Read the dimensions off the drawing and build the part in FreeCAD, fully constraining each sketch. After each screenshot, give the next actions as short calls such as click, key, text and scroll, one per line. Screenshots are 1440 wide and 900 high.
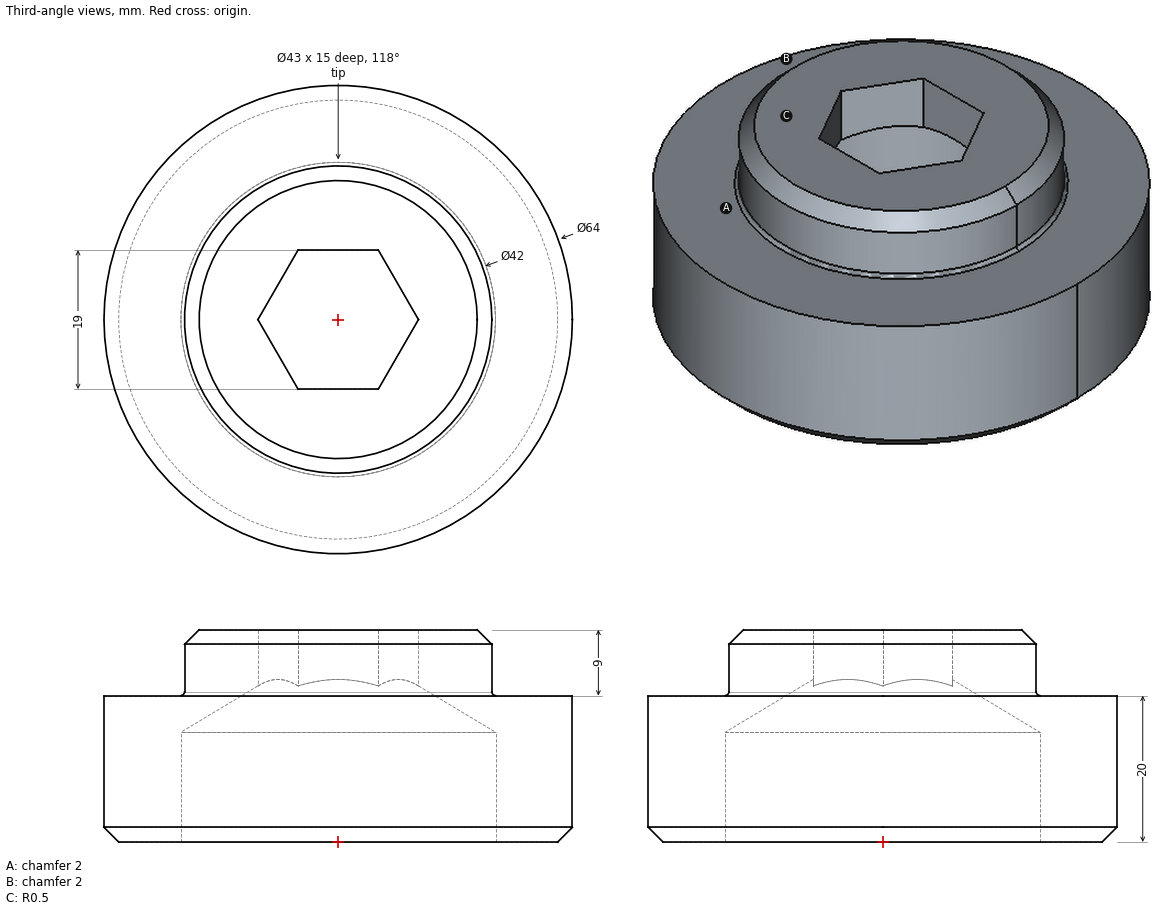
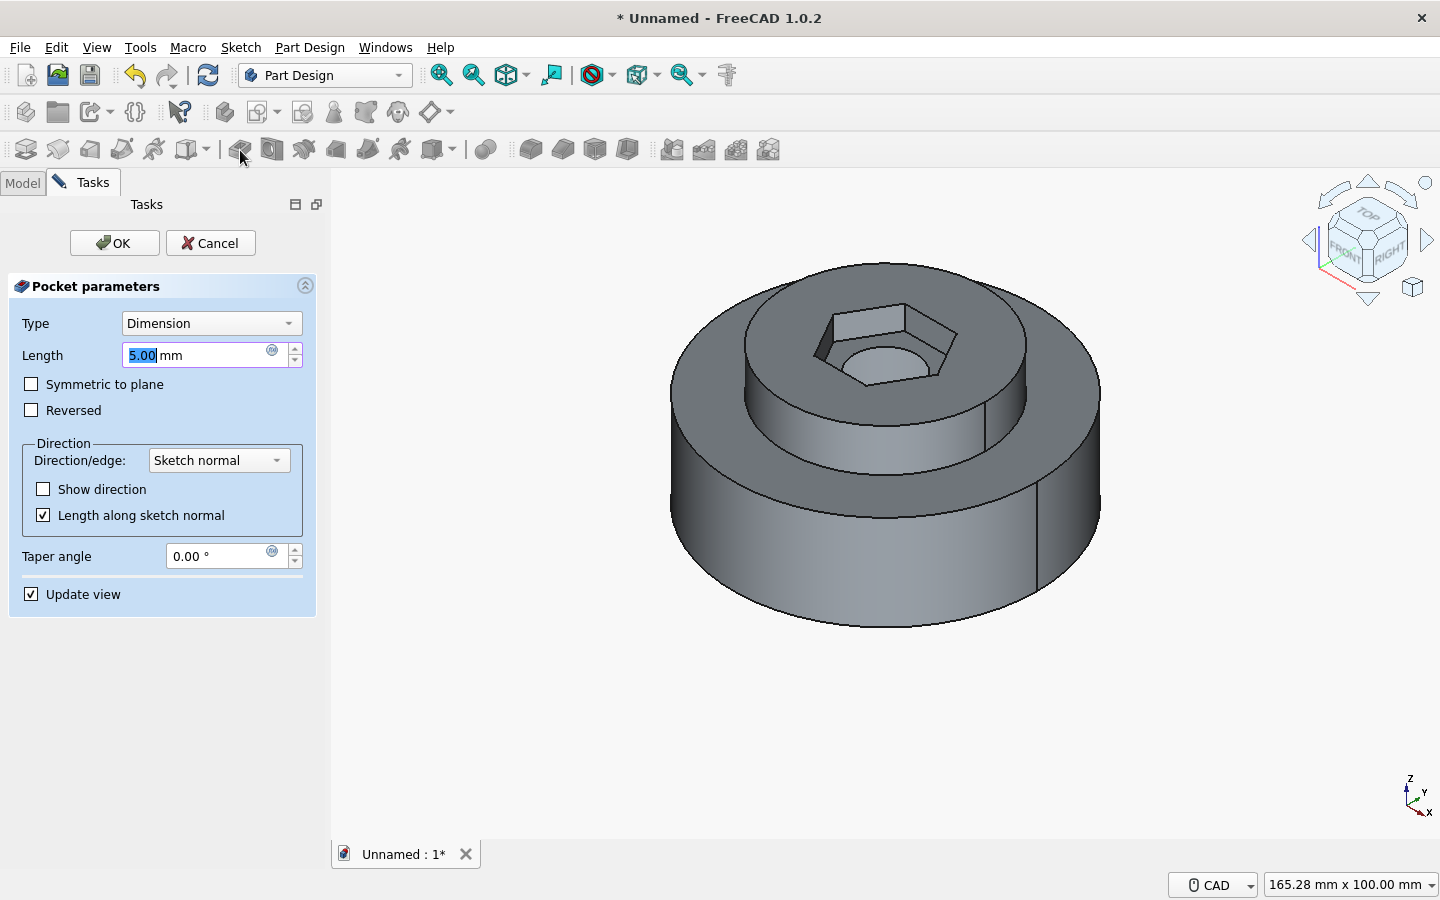
click(212, 324)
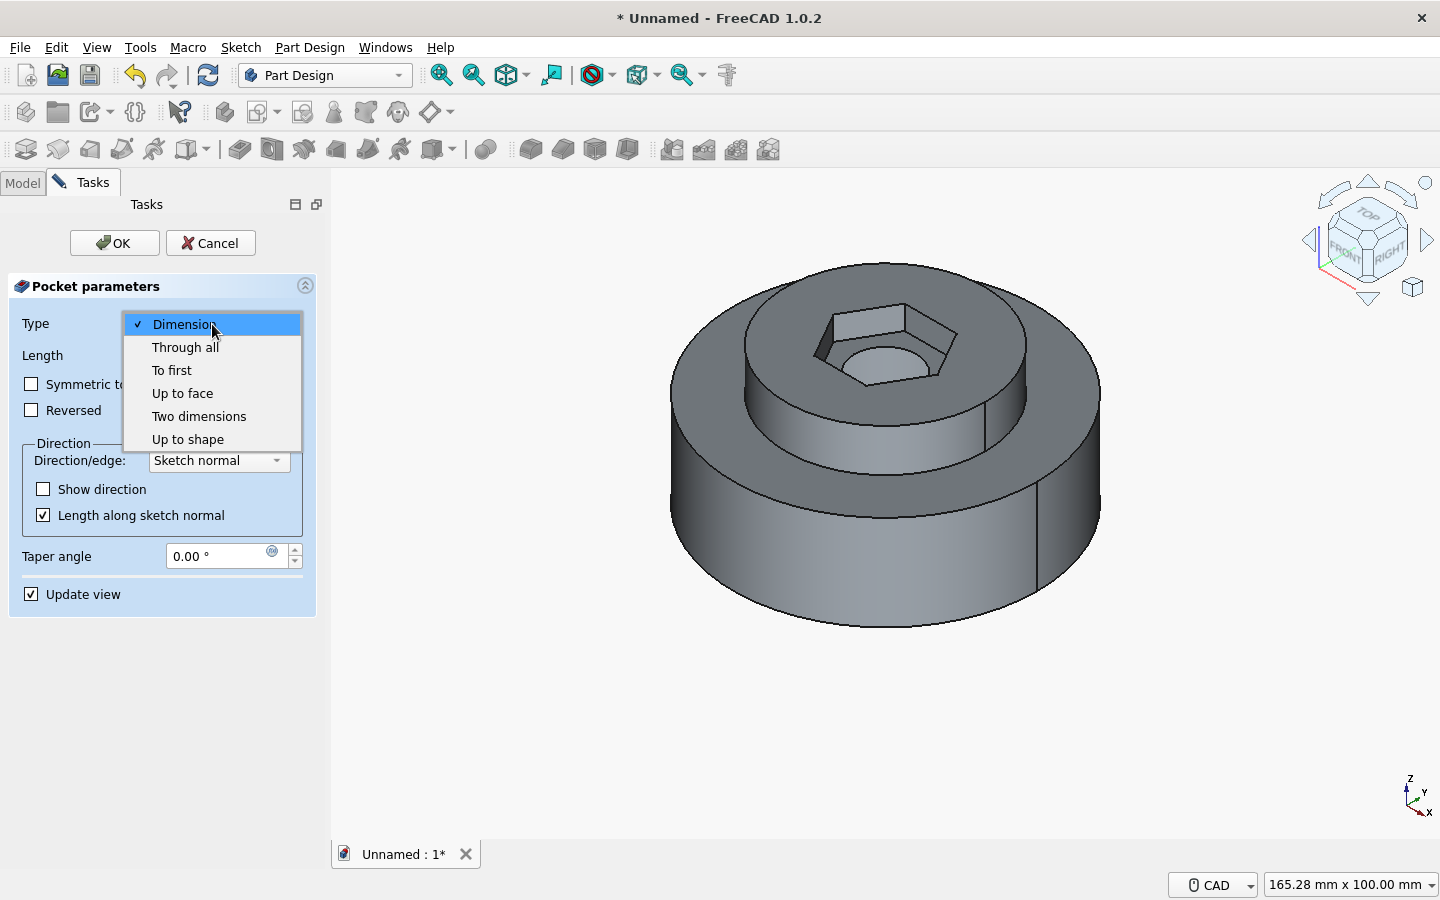
click(212, 348)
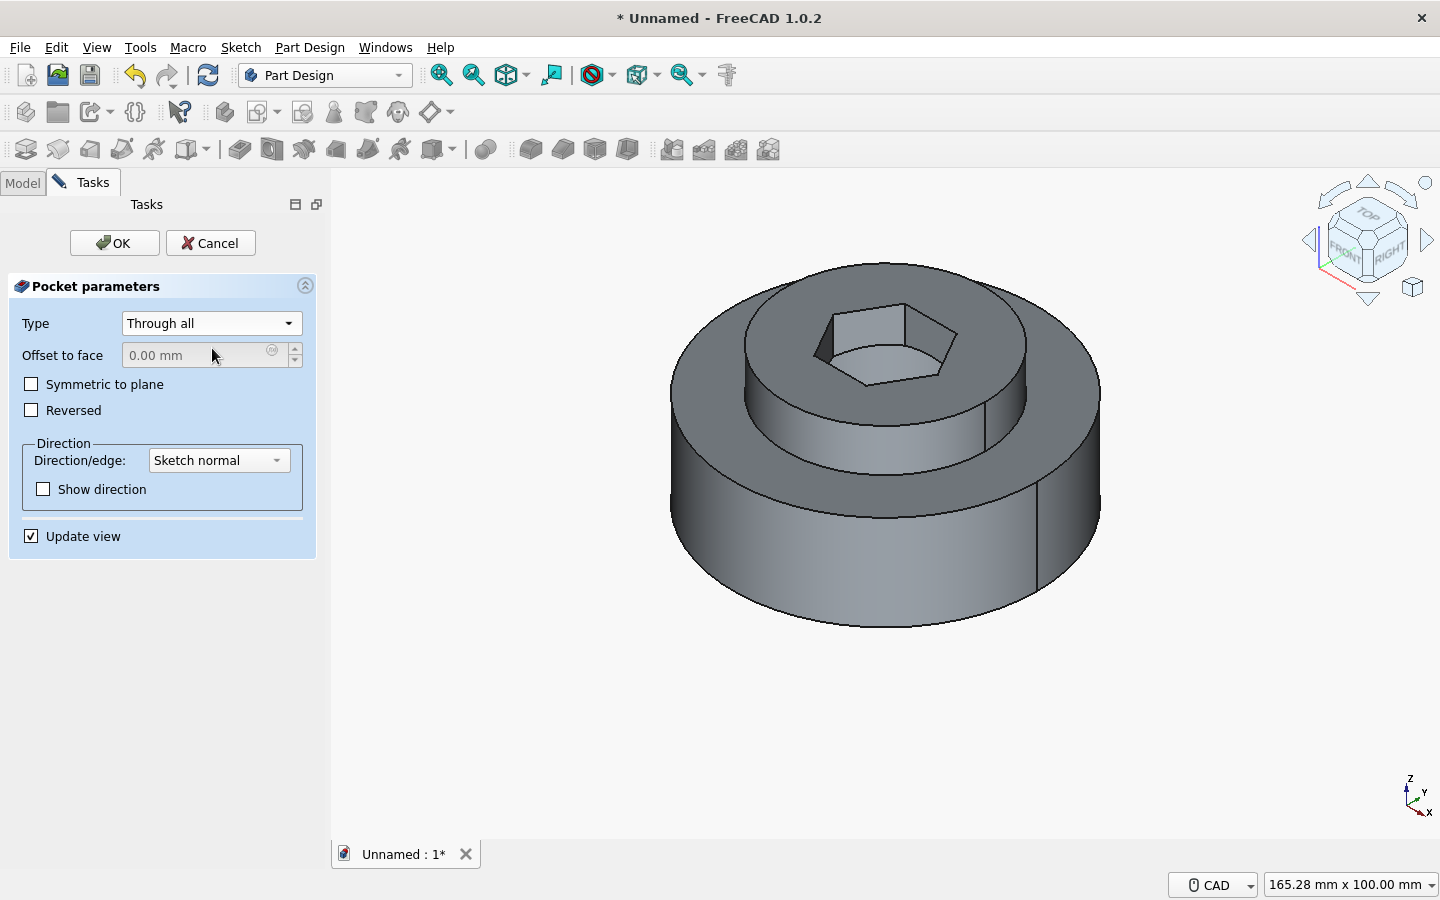
click(115, 243)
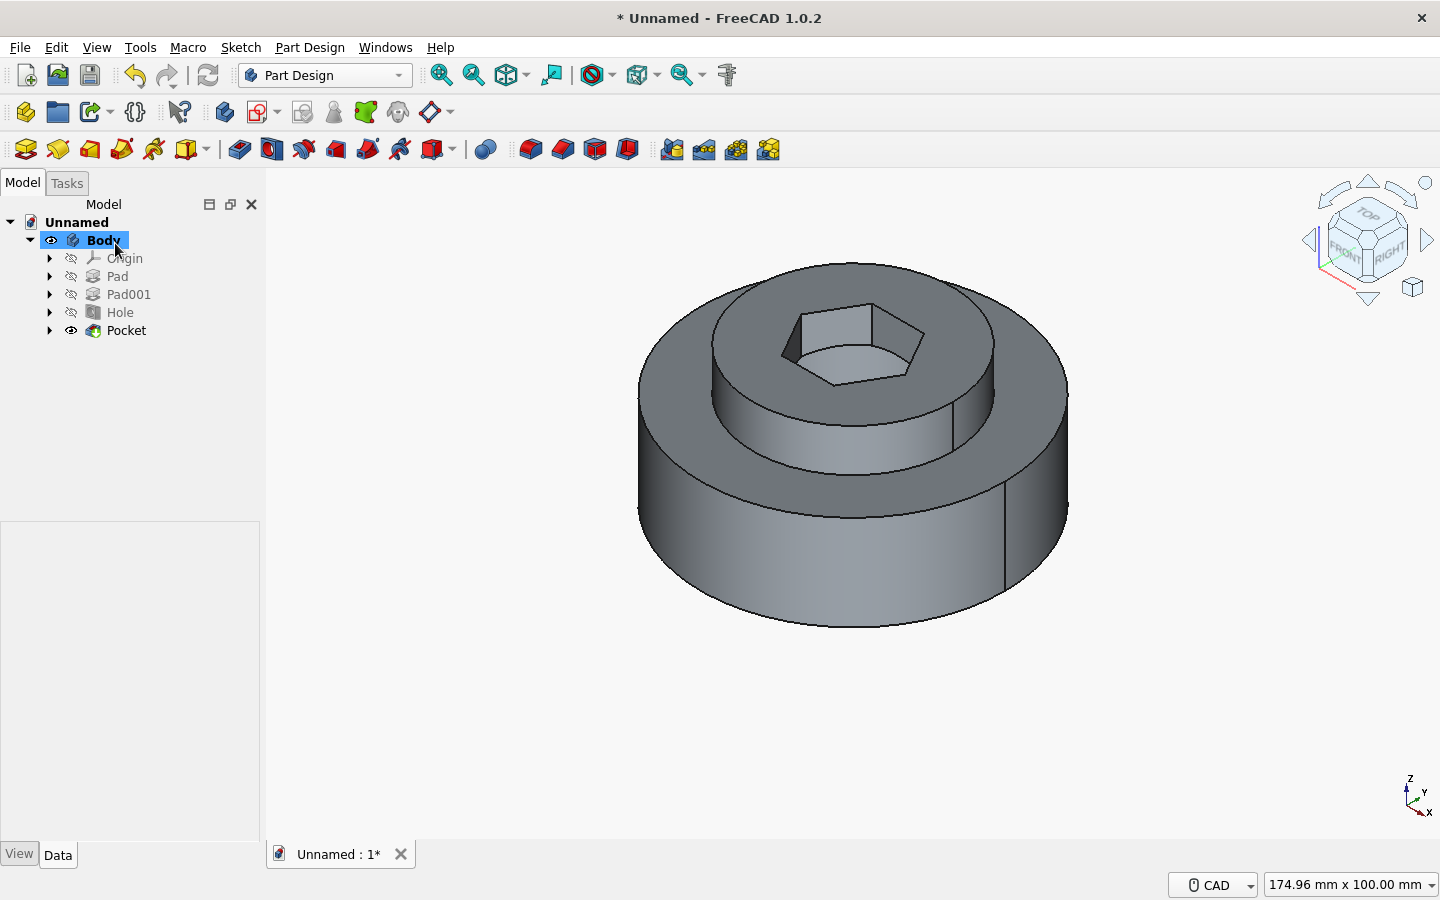
key(2)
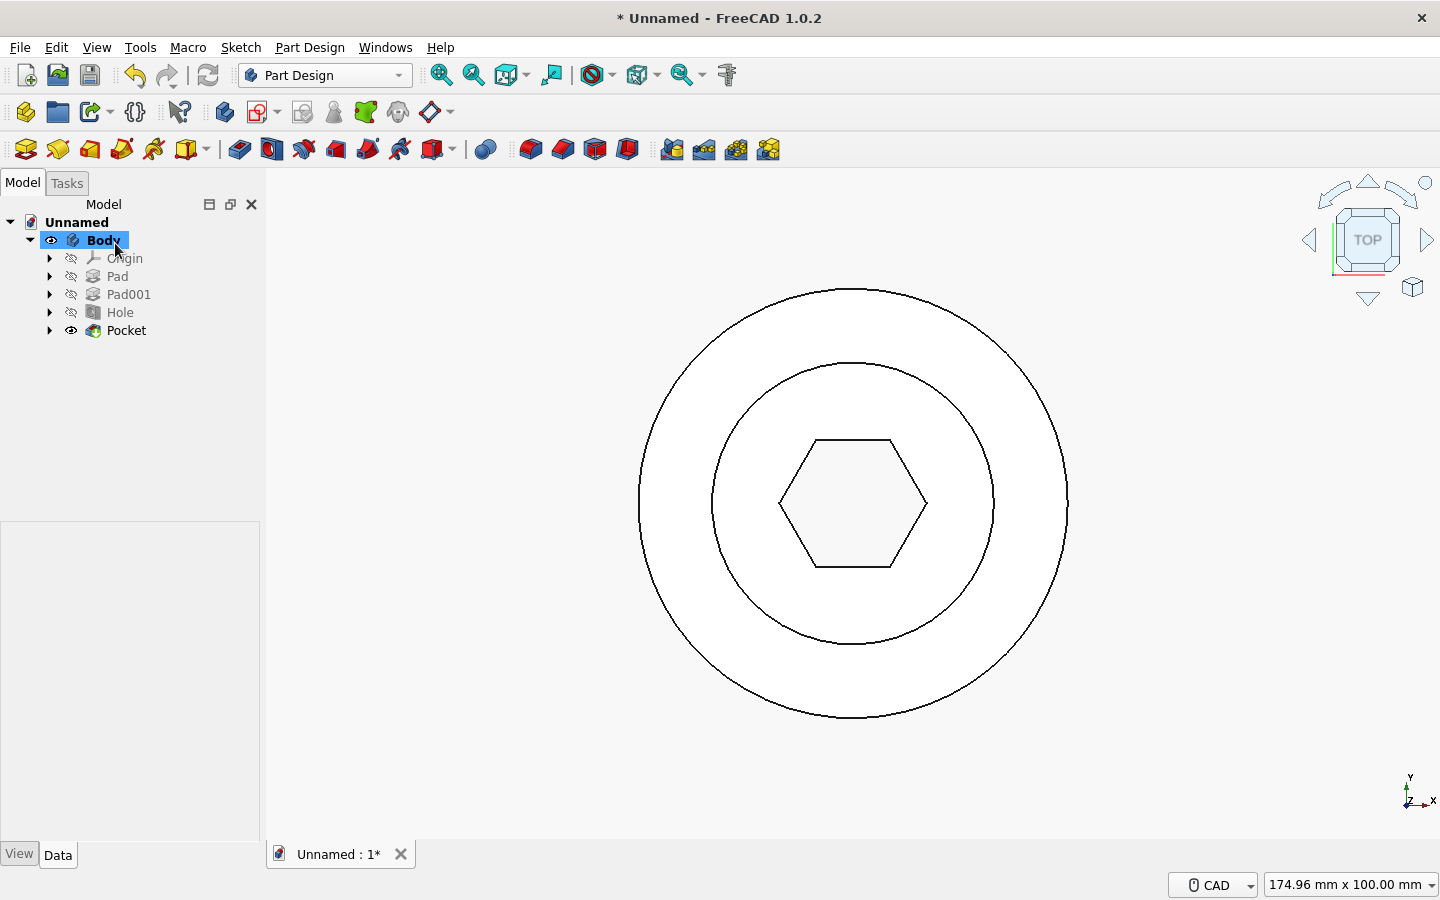
key(0)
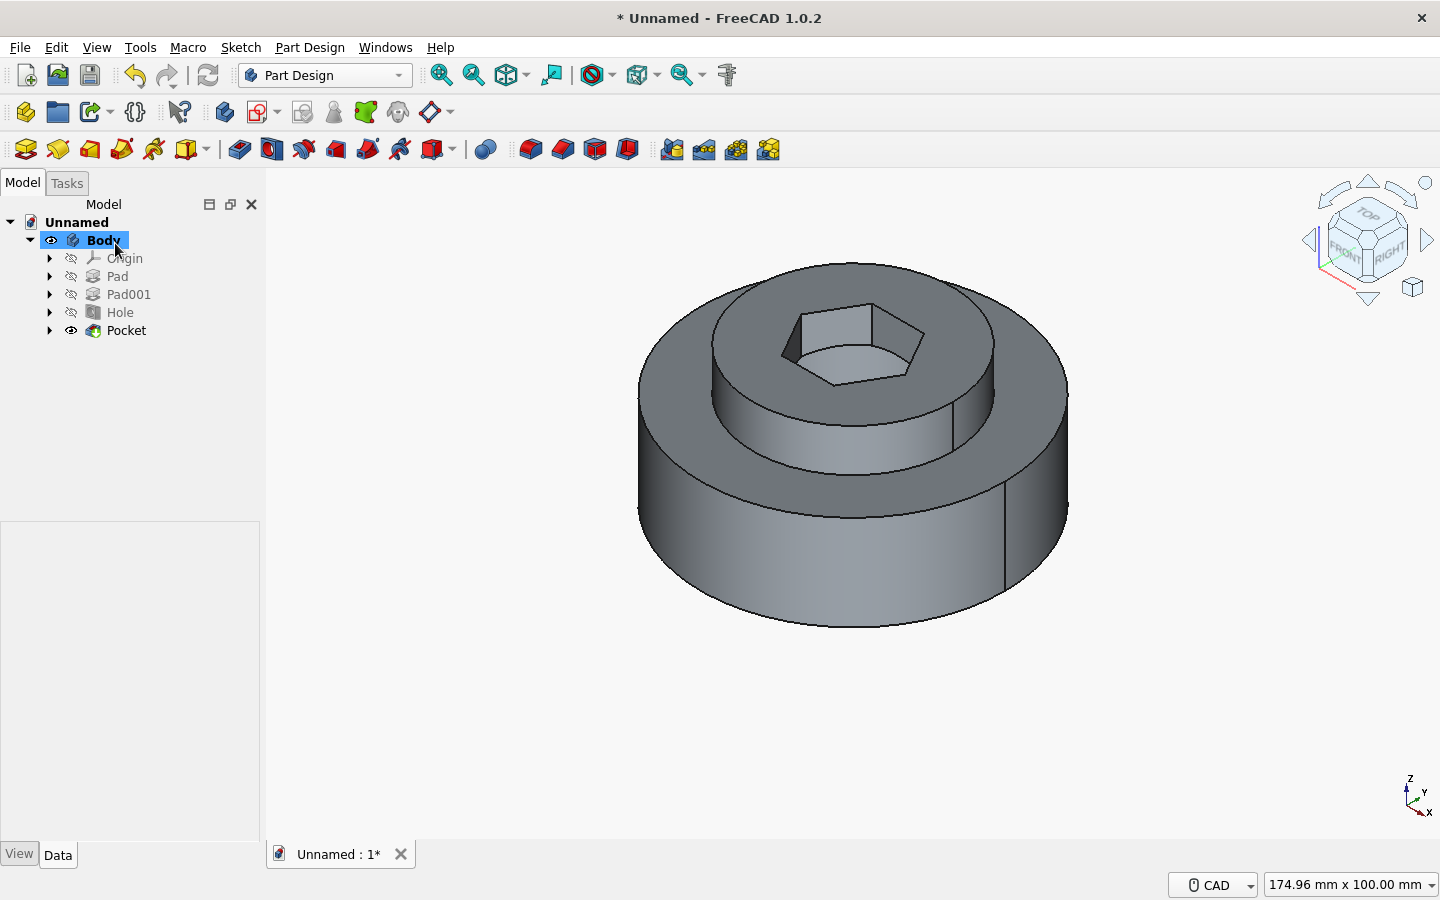
key(1)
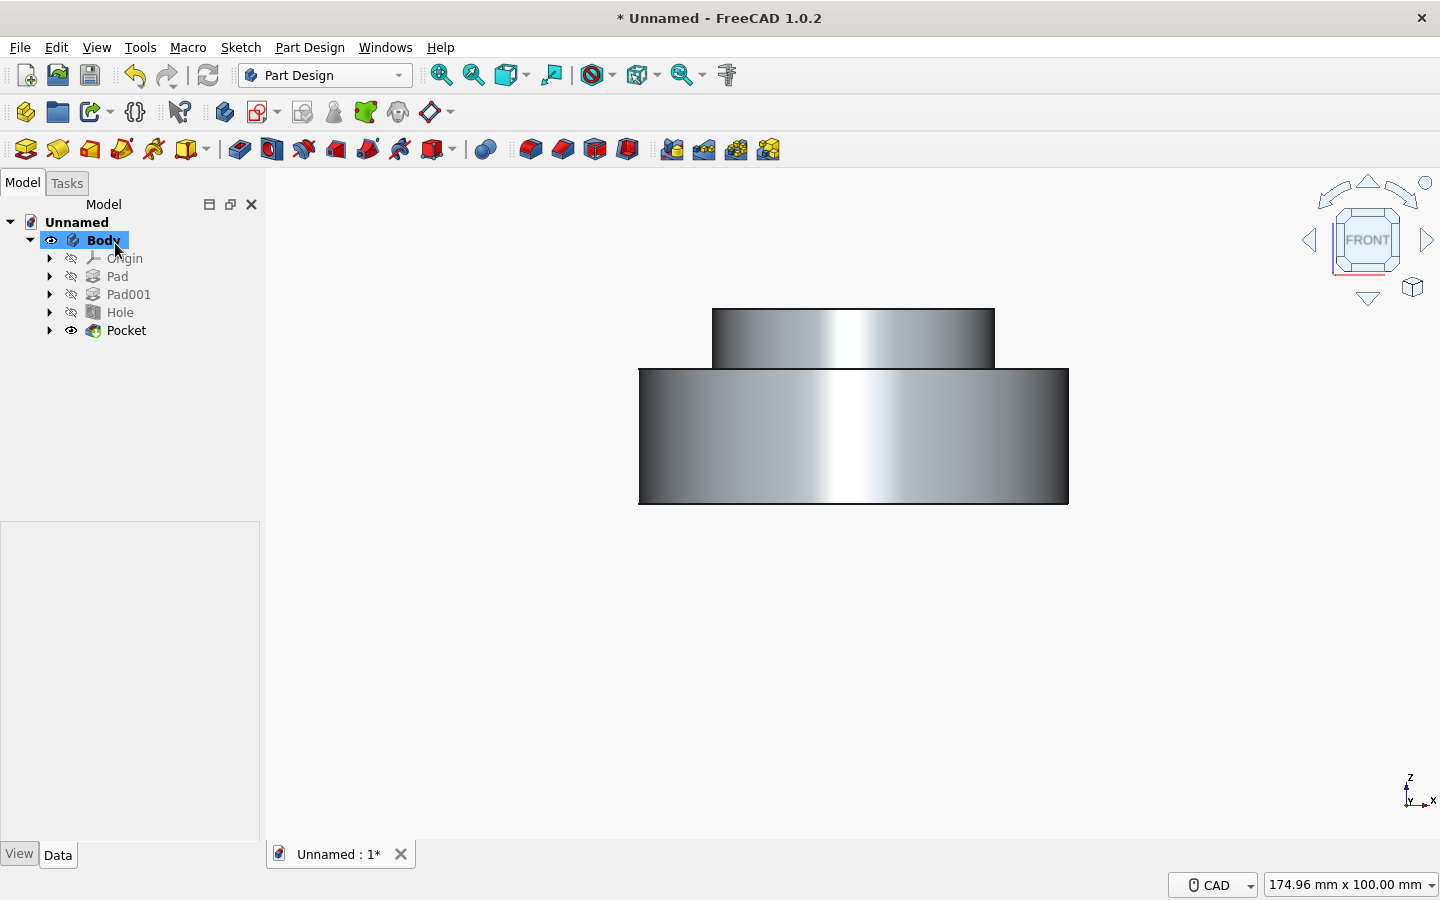
click(442, 76)